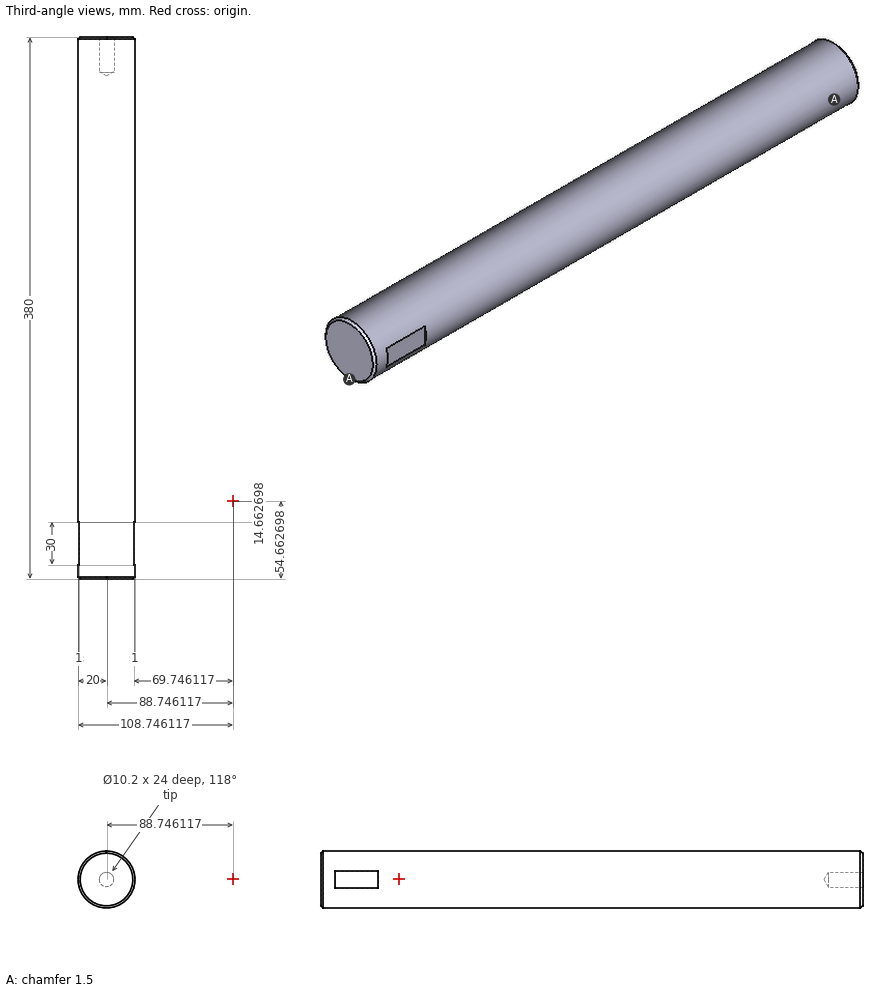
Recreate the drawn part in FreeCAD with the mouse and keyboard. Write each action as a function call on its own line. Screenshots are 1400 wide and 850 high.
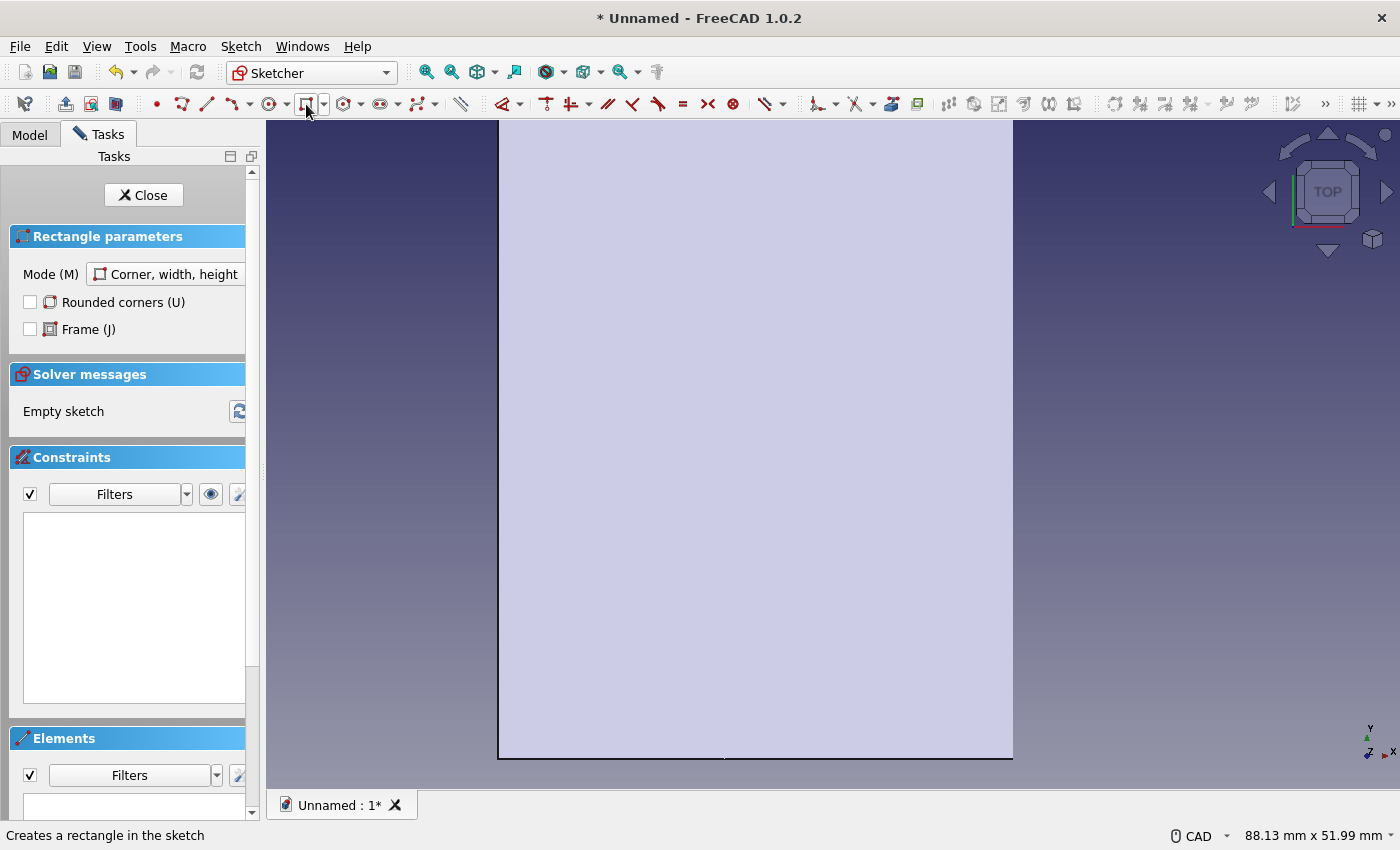
scroll(498, 244, up, 2)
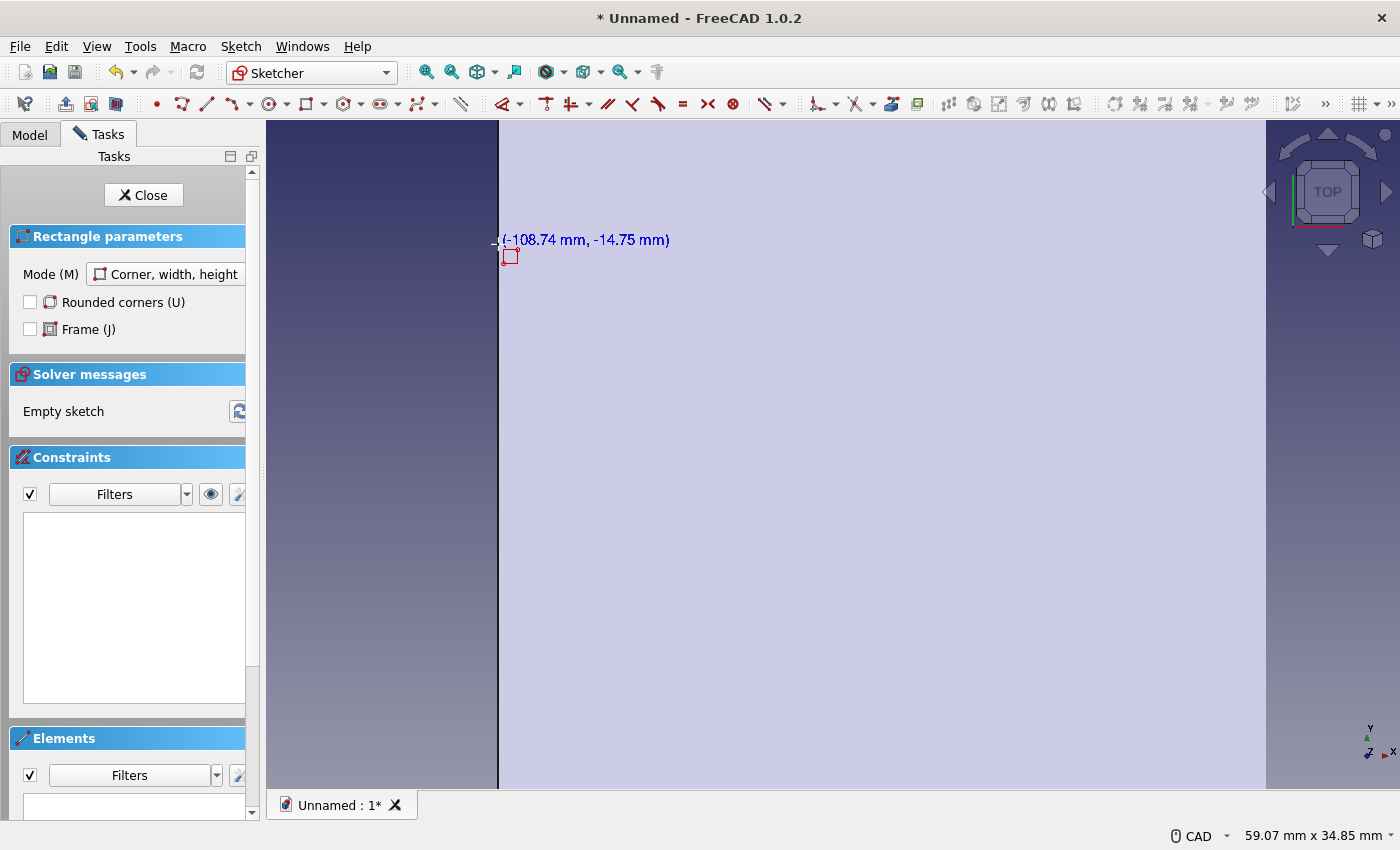
click(498, 244)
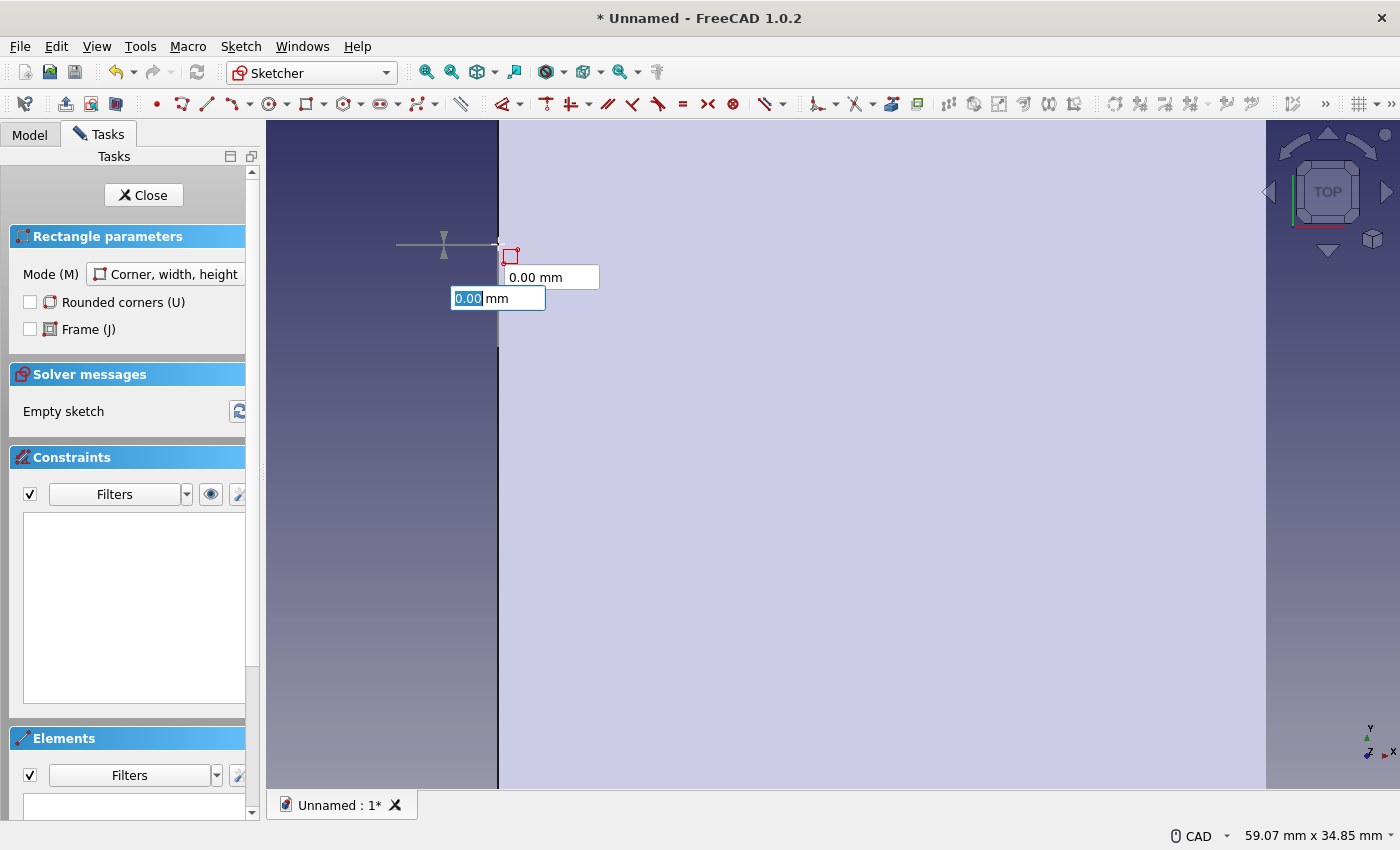
scroll(294, 148, down, 1)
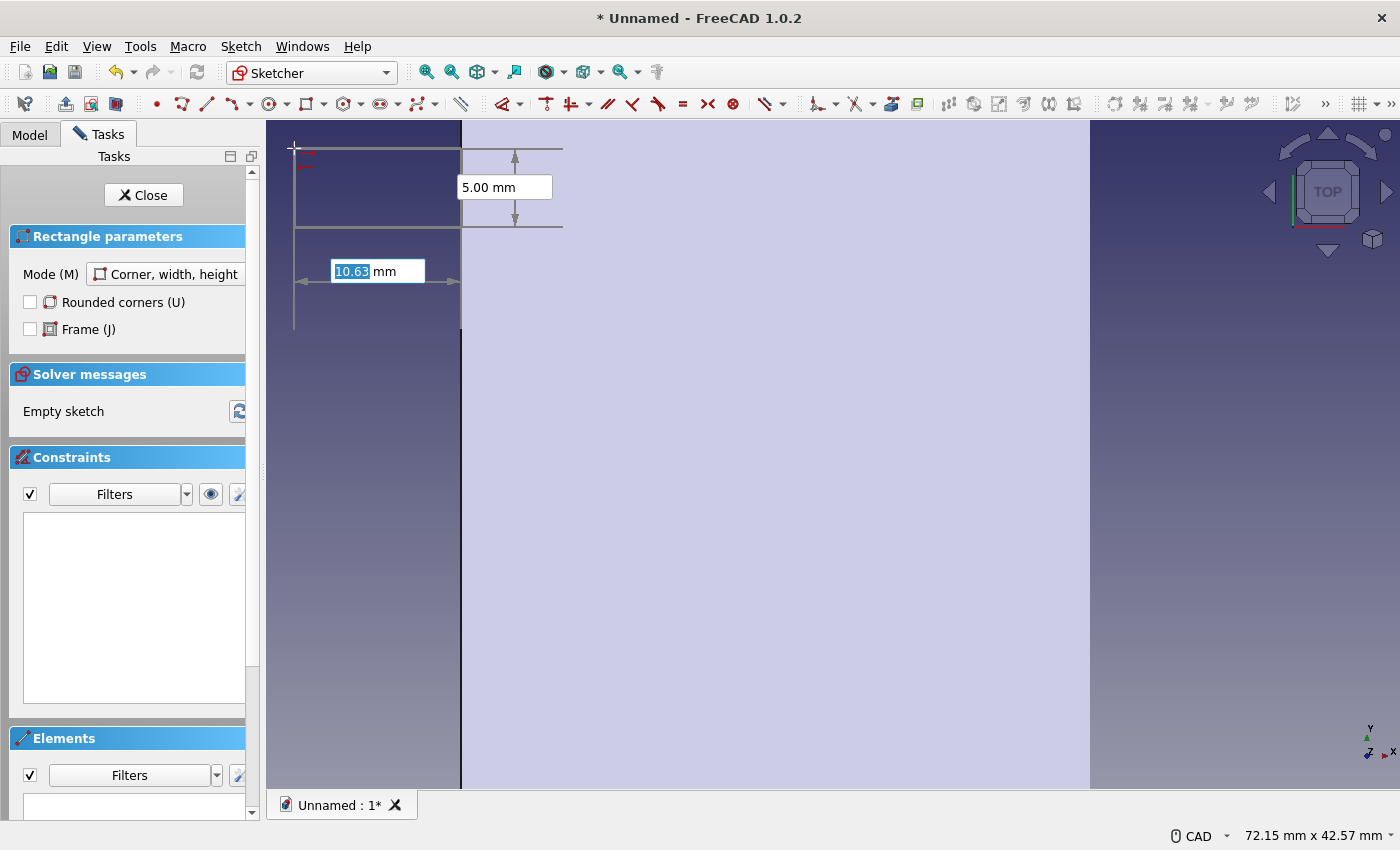
click(477, 698)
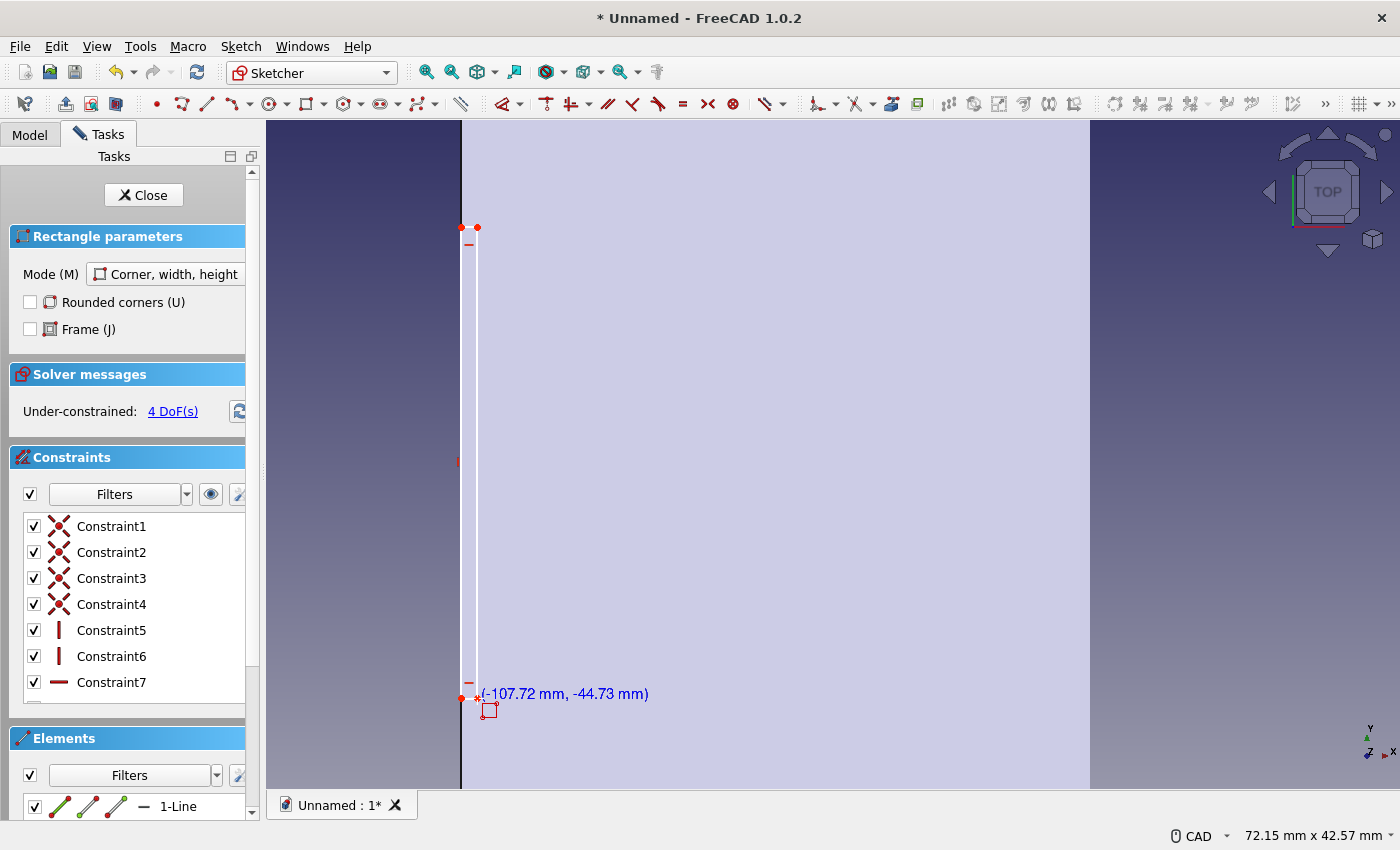
click(1074, 226)
move(1090, 698)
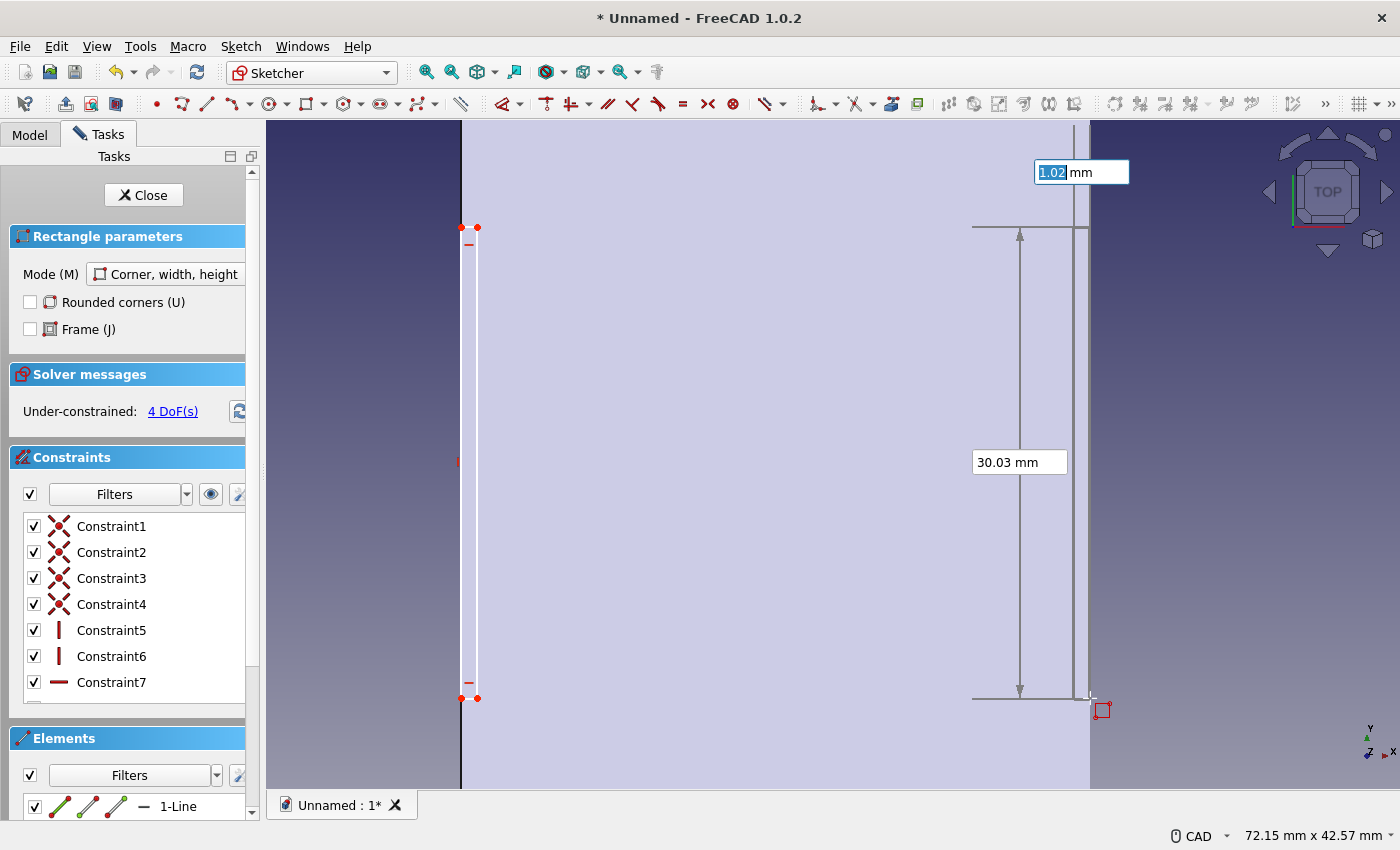
text(1)
key(Tab)
text(30)
key(Return)
key(Escape)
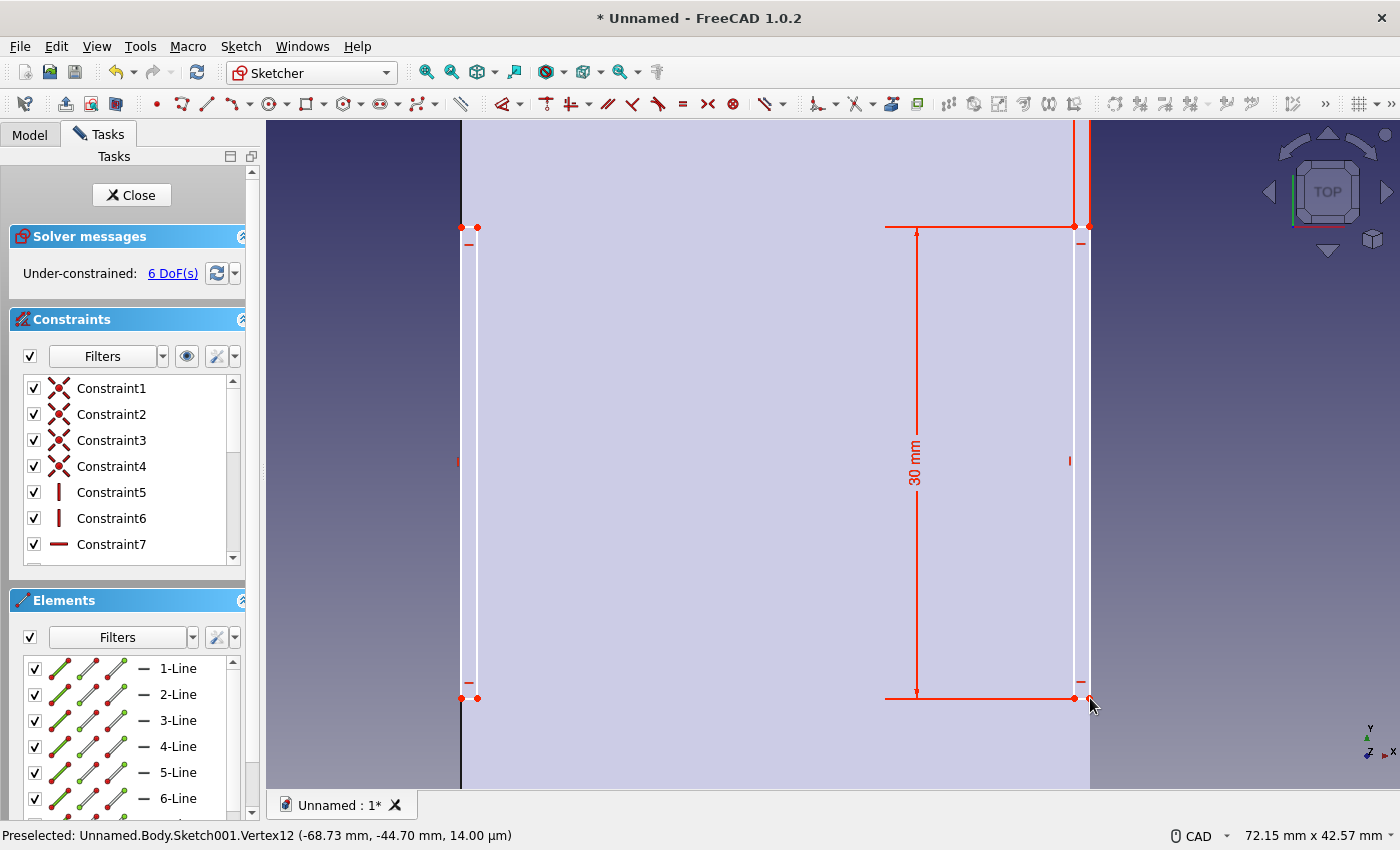
click(502, 104)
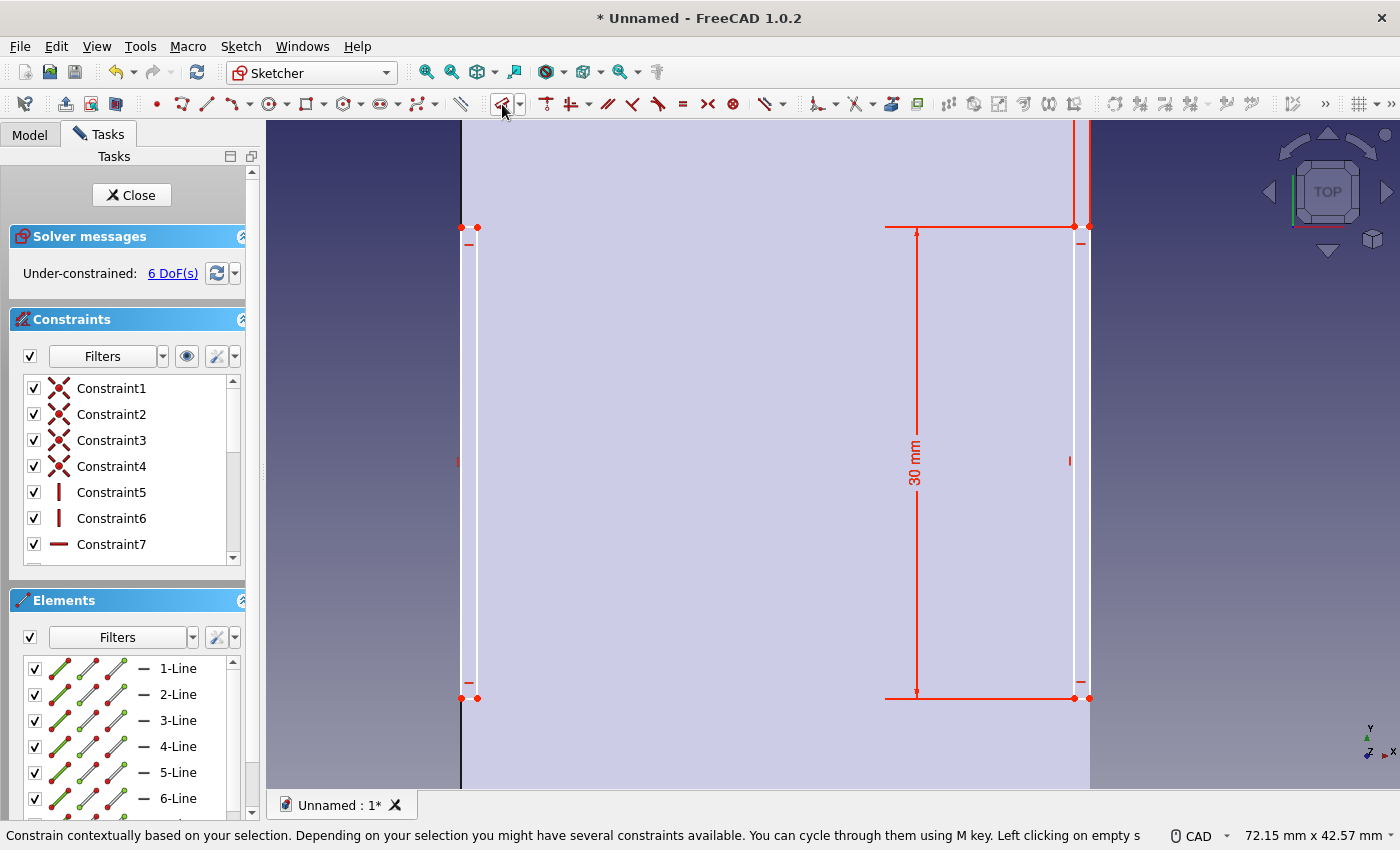
scroll(469, 699, up, 5)